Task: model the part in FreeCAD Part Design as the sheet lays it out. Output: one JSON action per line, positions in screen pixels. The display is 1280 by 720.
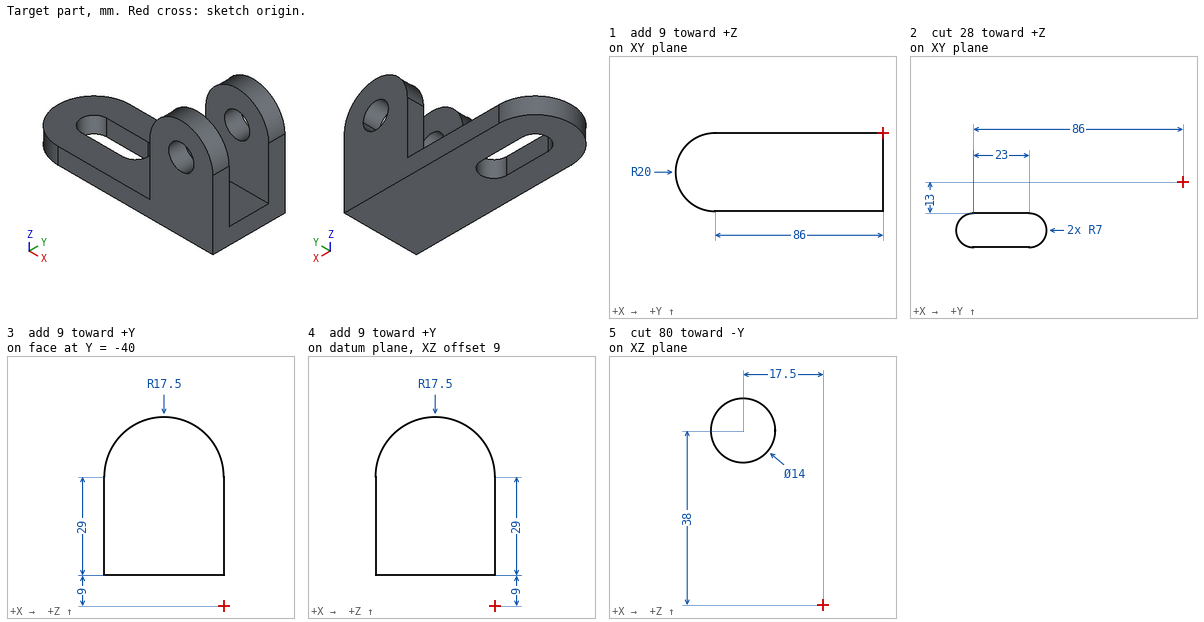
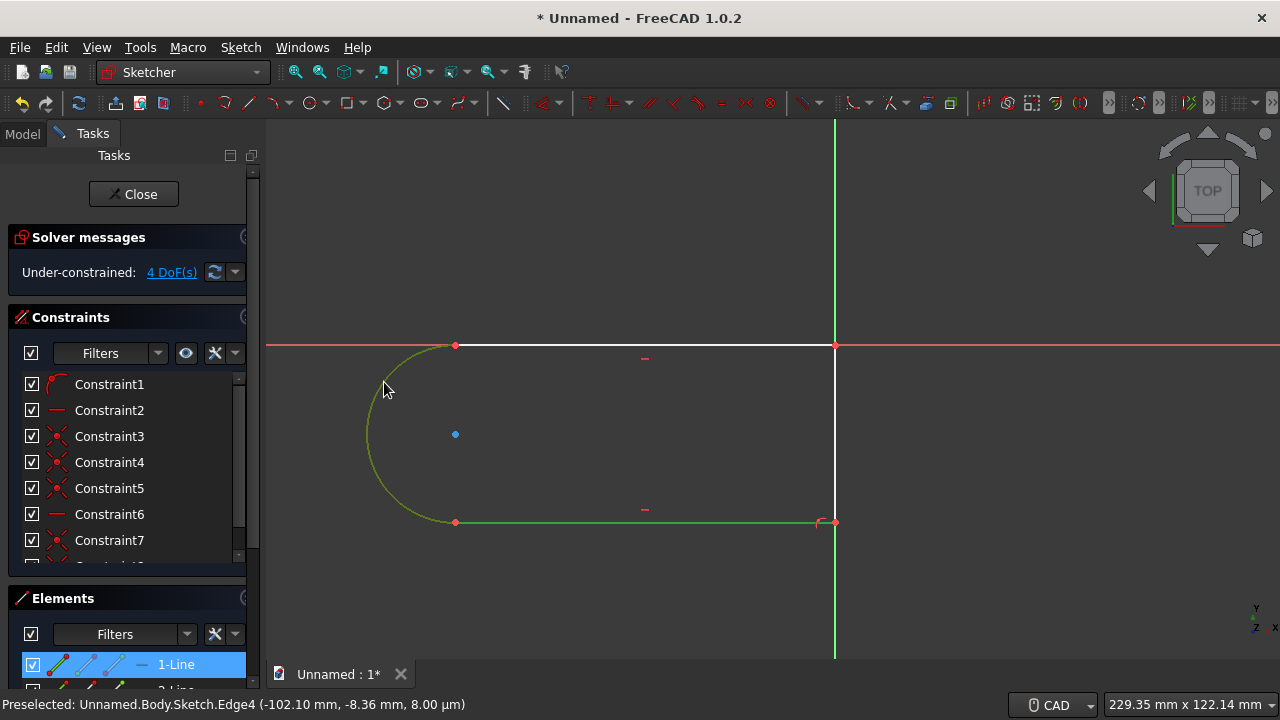
{"action": "left_click", "coordinate": [698, 104]}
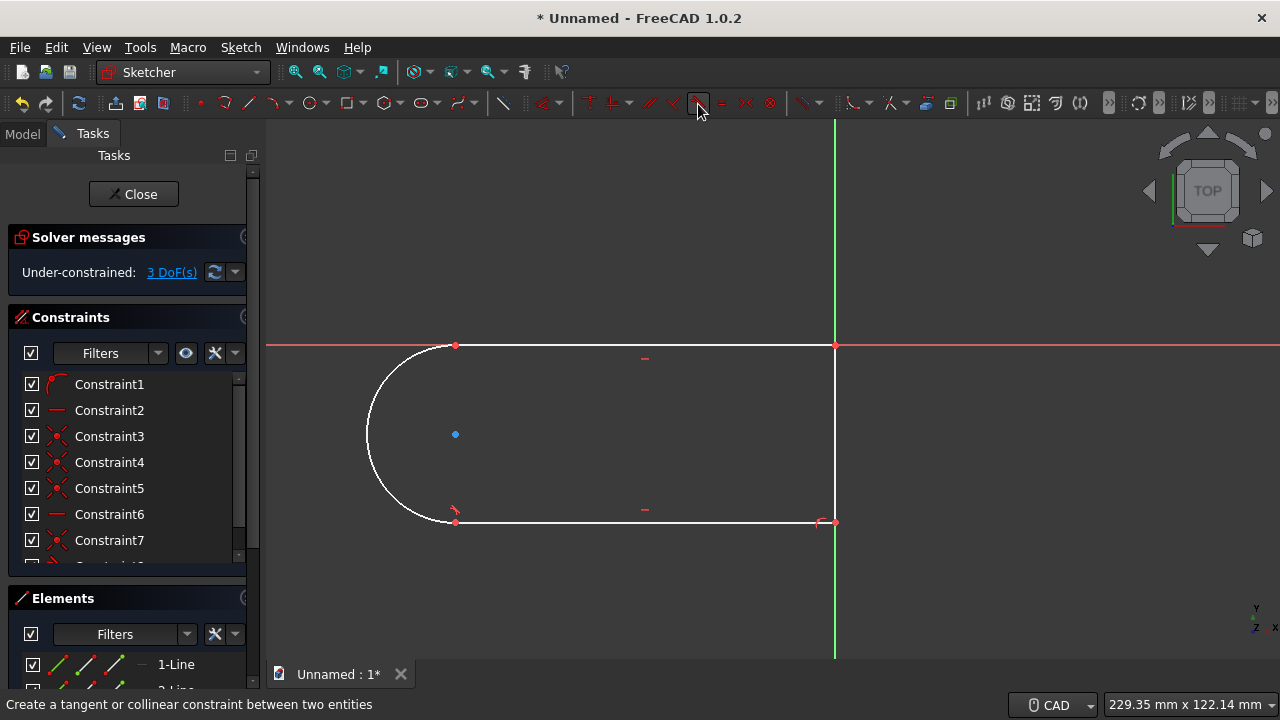
{"action": "left_click", "coordinate": [721, 345]}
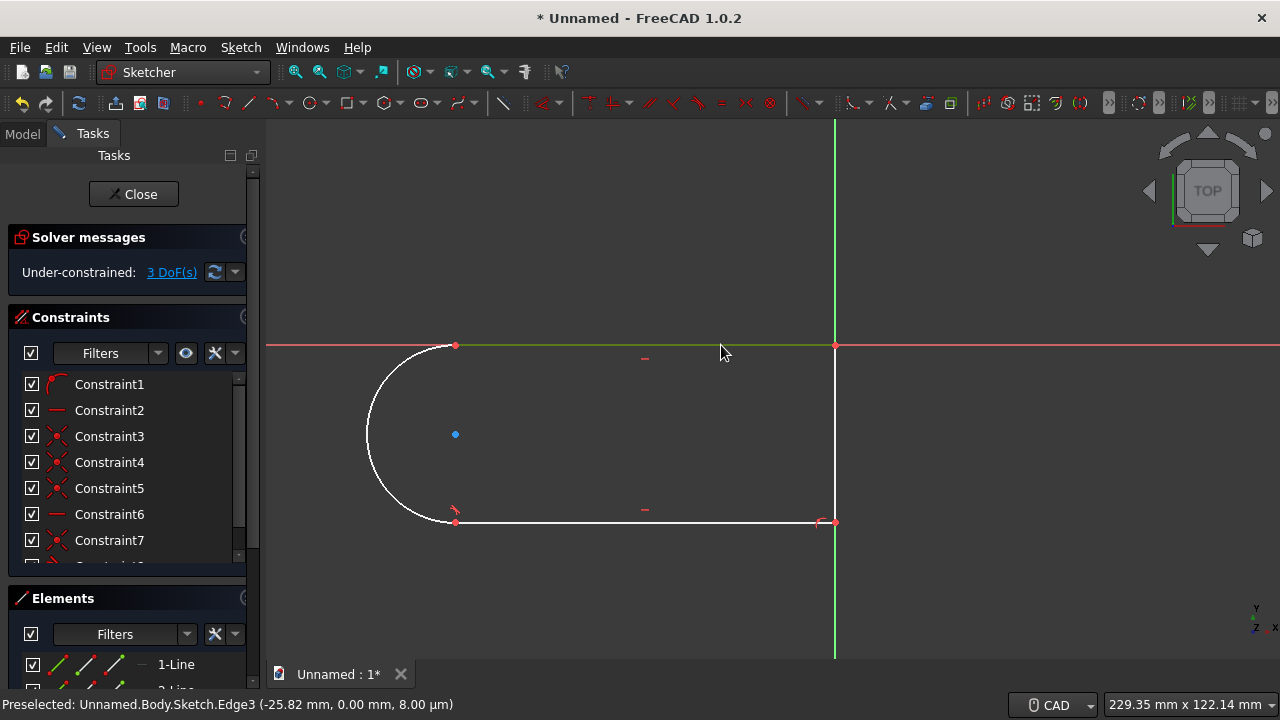
{"action": "left_click", "coordinate": [384, 382]}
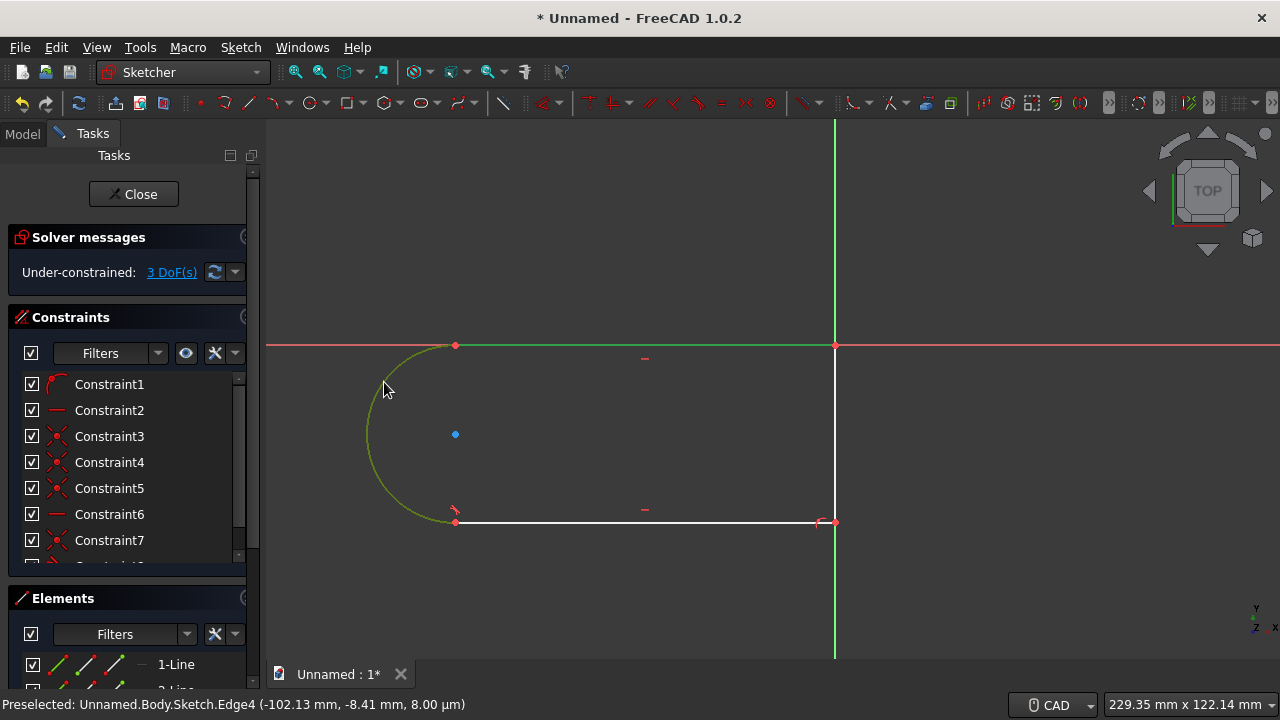
{"action": "left_click", "coordinate": [698, 104]}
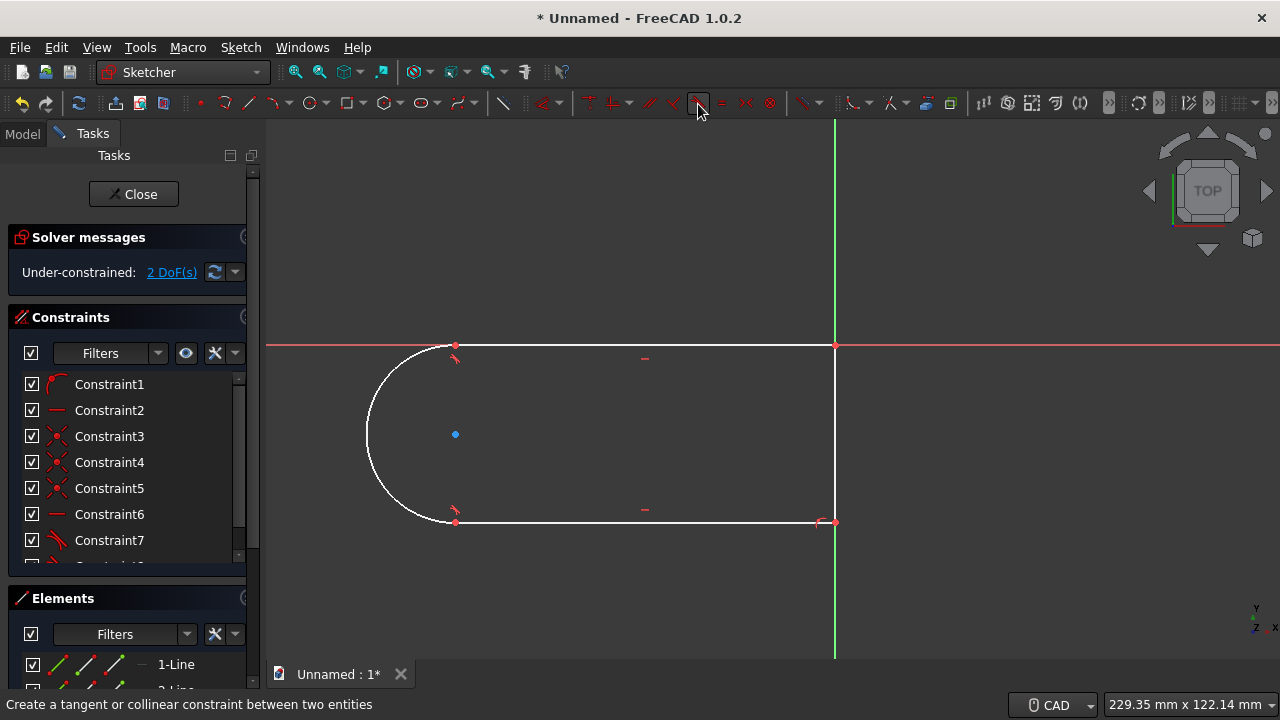
{"action": "left_click", "coordinate": [542, 104]}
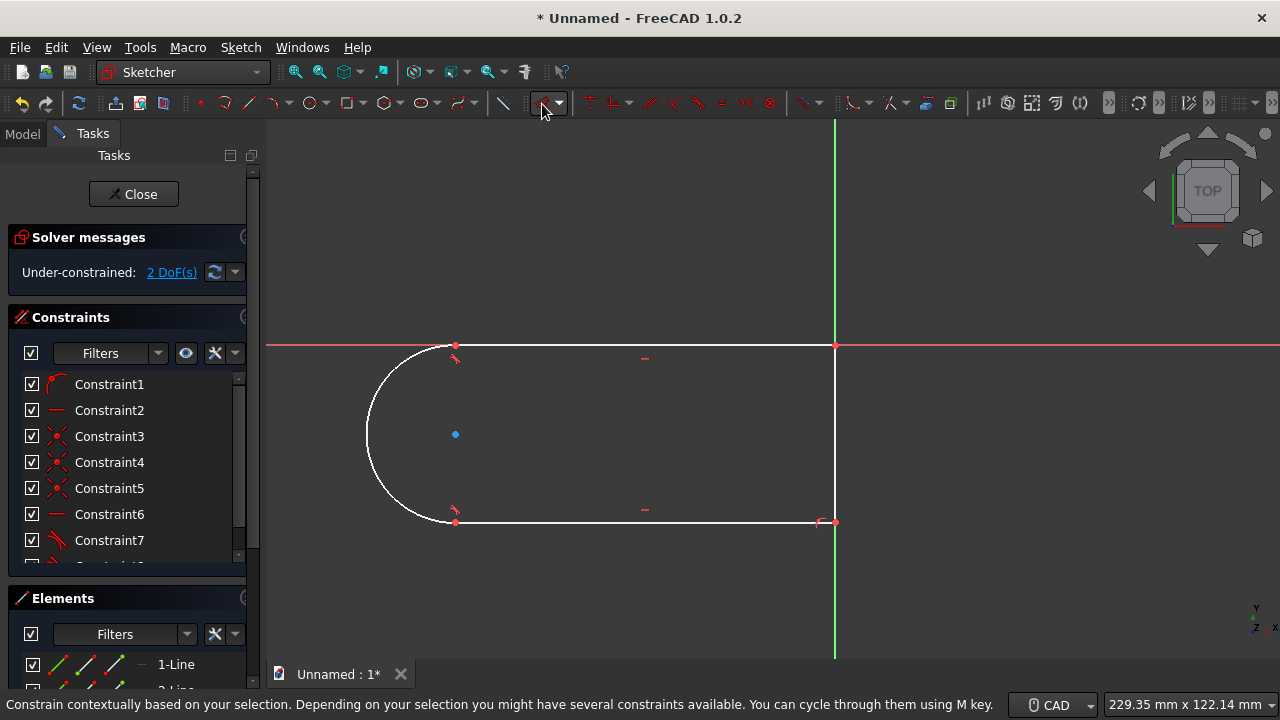
{"action": "left_click", "coordinate": [383, 382]}
{"action": "left_click", "coordinate": [357, 363]}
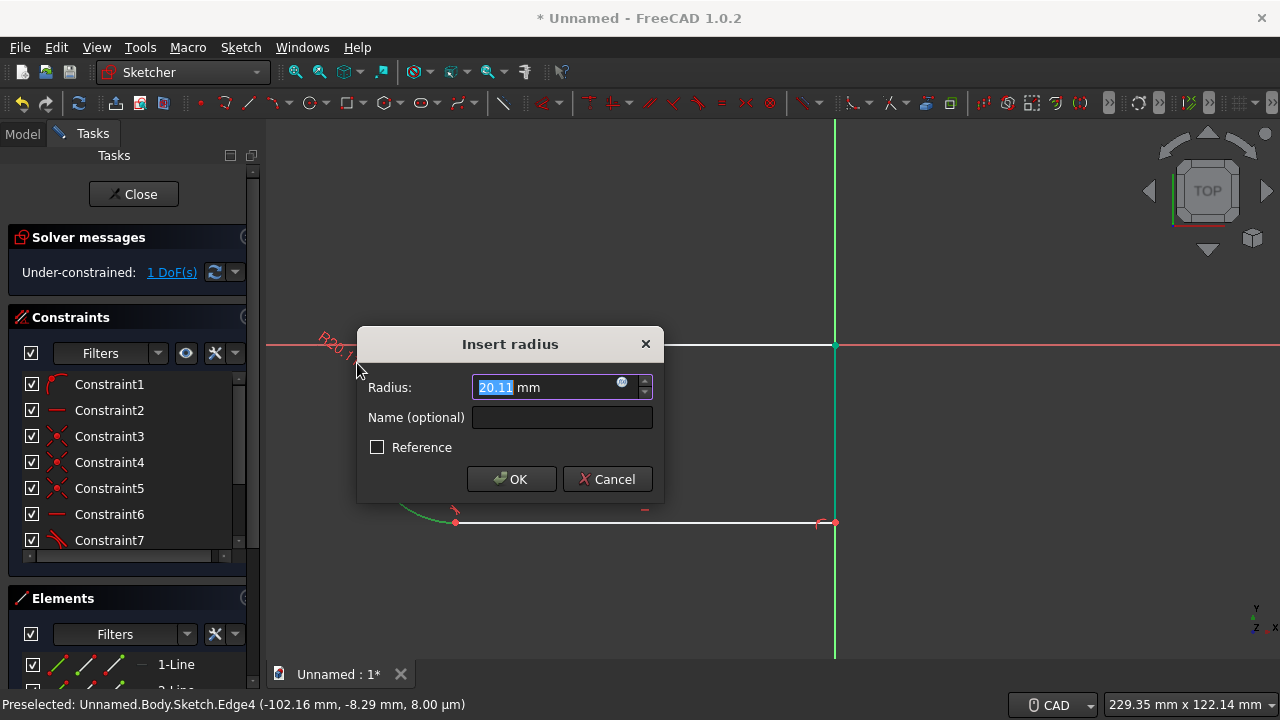
{"action": "type", "text": "20"}
{"action": "key", "text": "Return"}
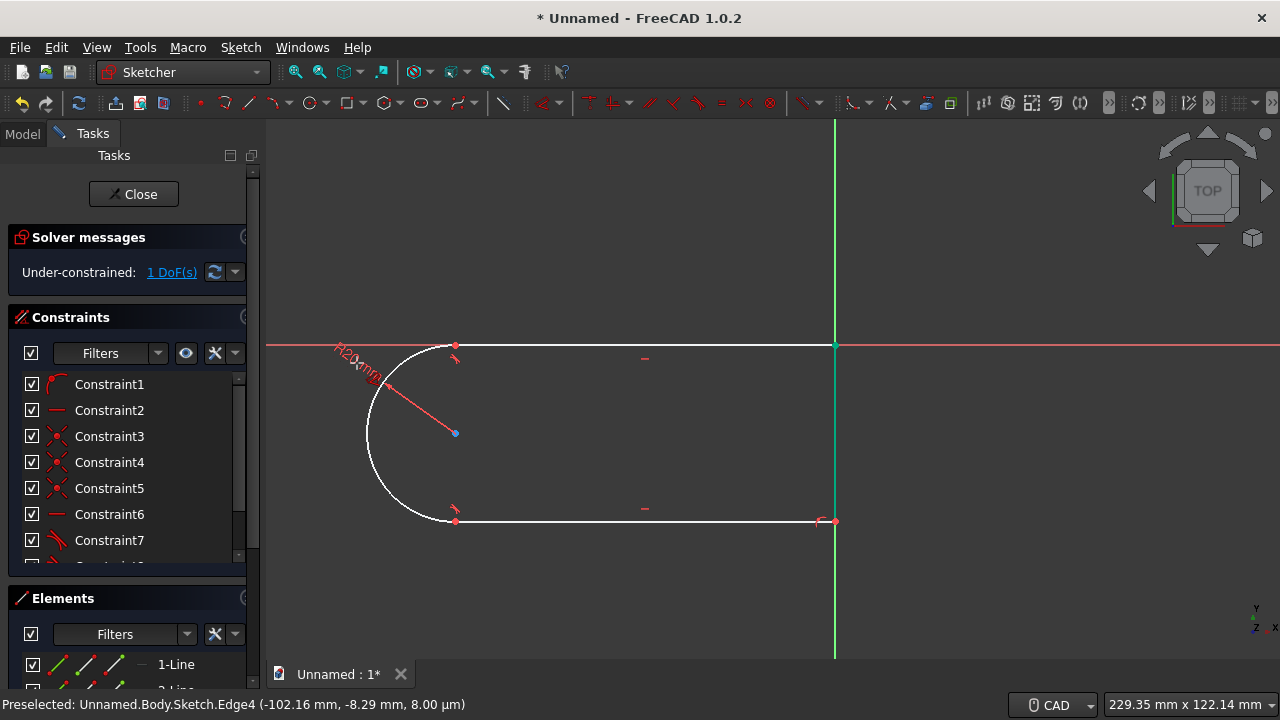
{"action": "left_click", "coordinate": [569, 522]}
{"action": "left_click", "coordinate": [645, 556]}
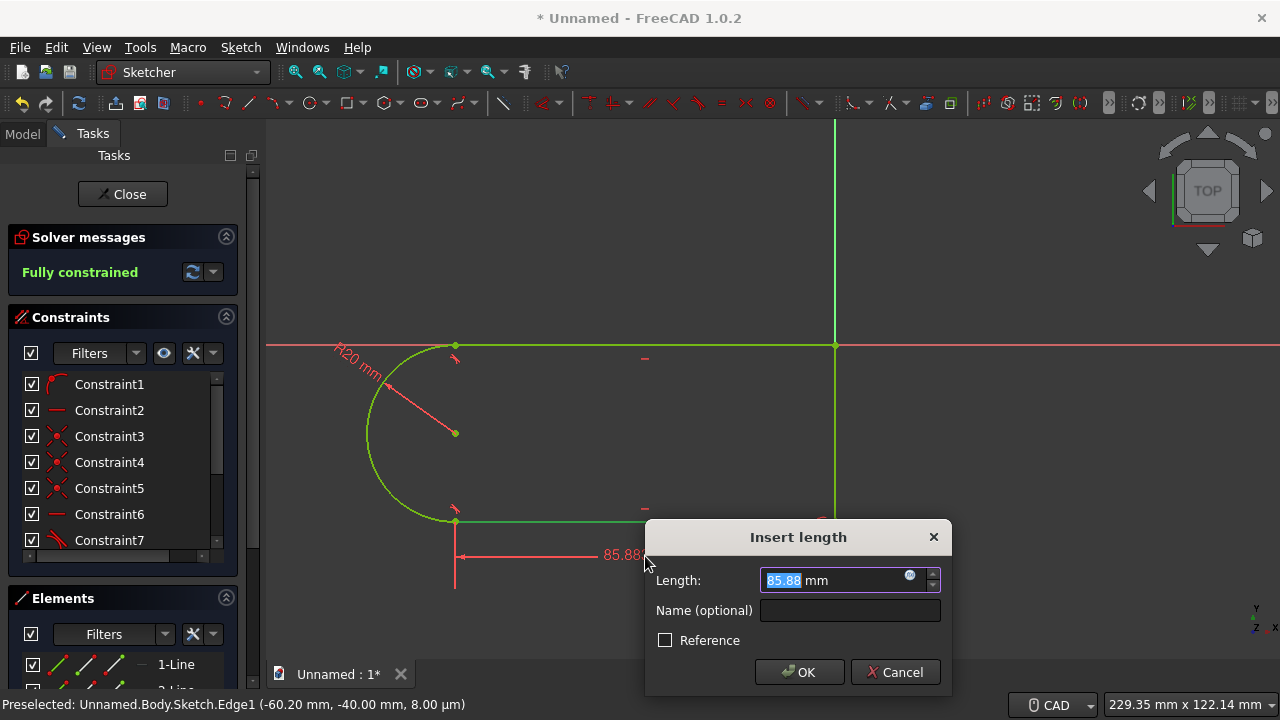
{"action": "type", "text": "86"}
{"action": "key", "text": "Return"}
{"action": "key", "text": "Escape"}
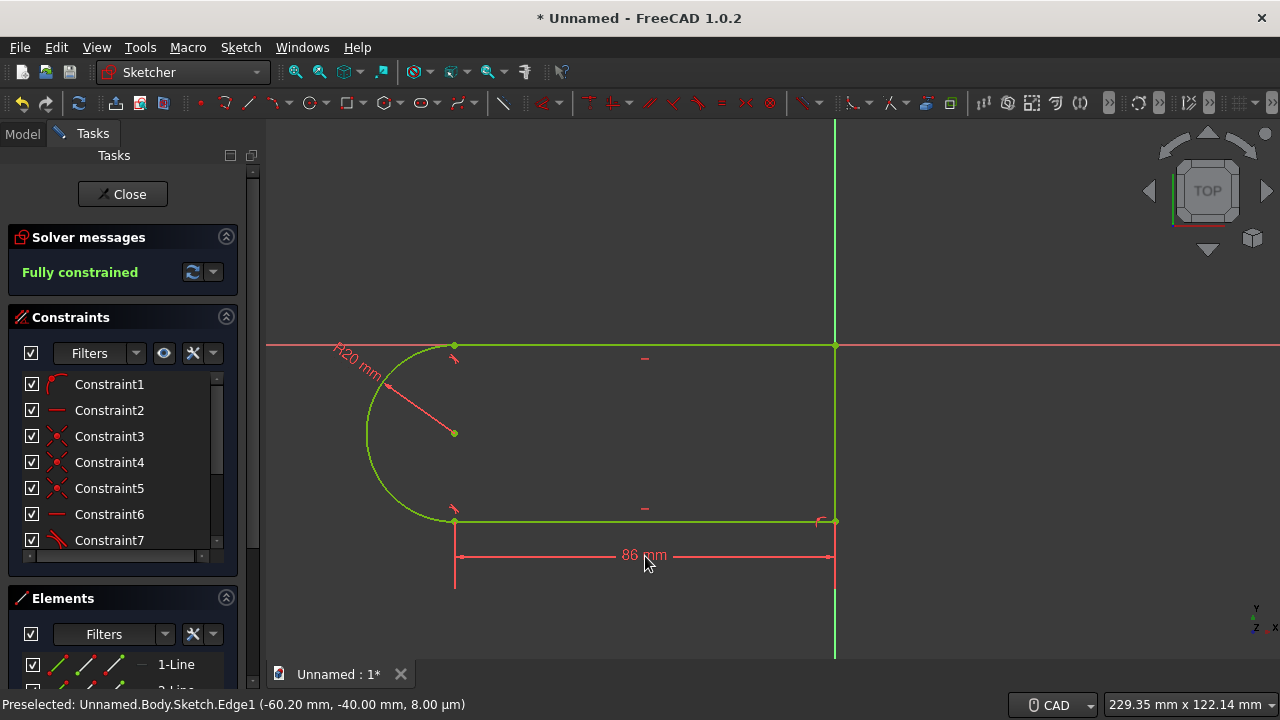
{"action": "left_click", "coordinate": [123, 194]}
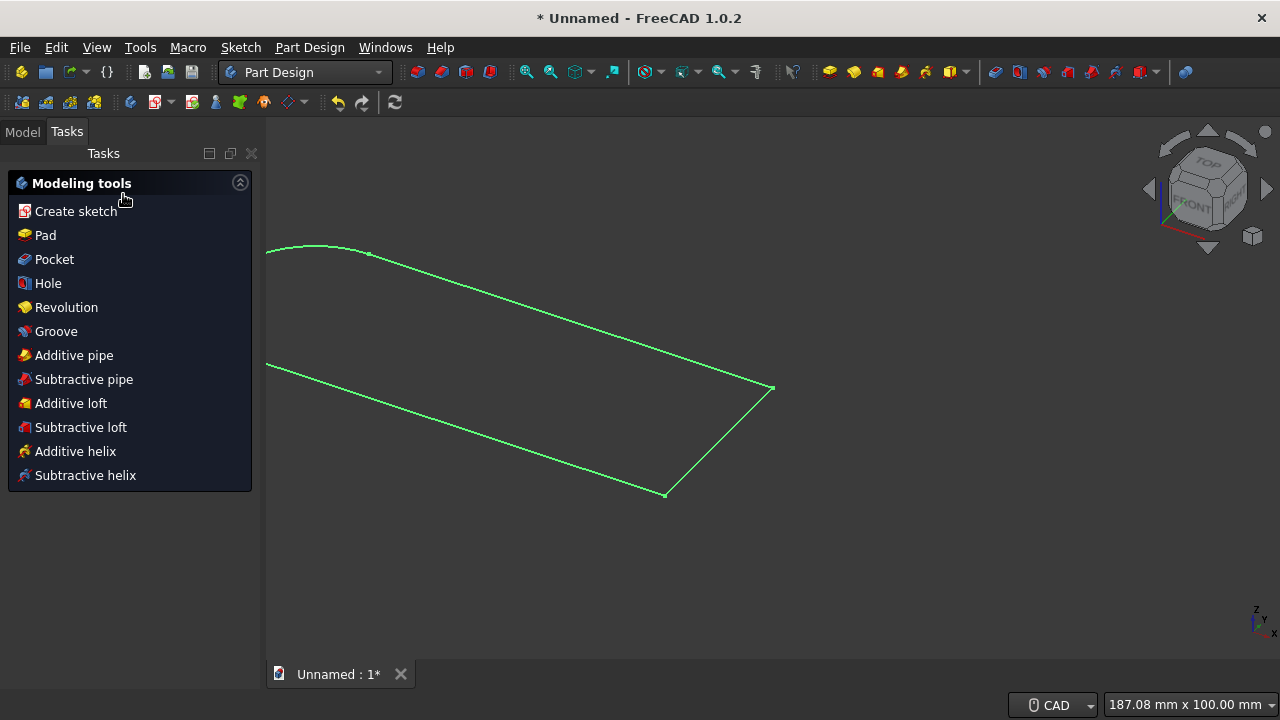
{"action": "left_click", "coordinate": [830, 72]}